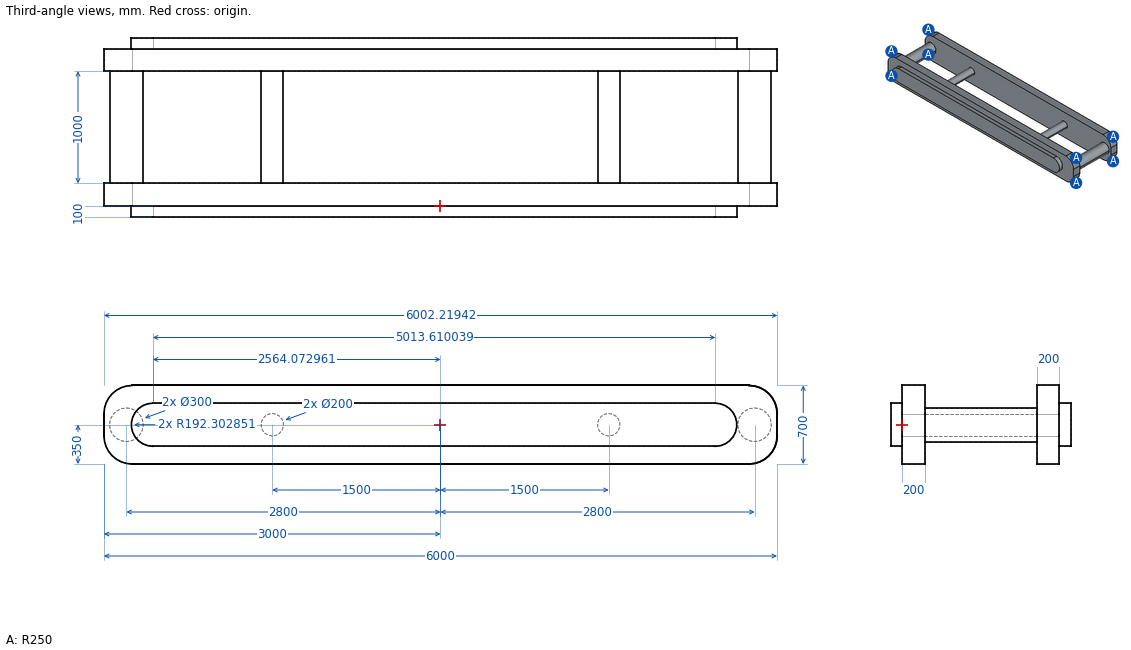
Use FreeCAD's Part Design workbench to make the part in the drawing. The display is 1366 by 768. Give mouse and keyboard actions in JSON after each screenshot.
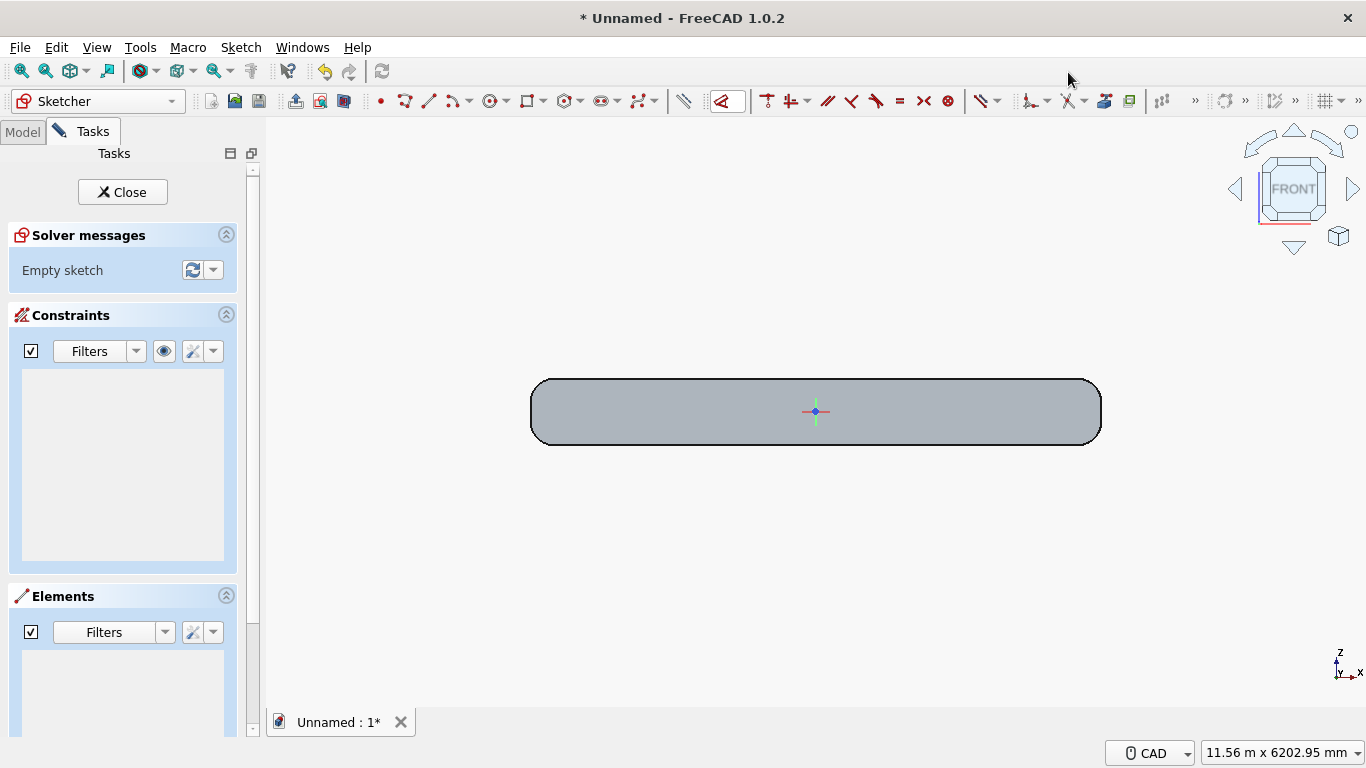
{"action": "left_click", "coordinate": [602, 102]}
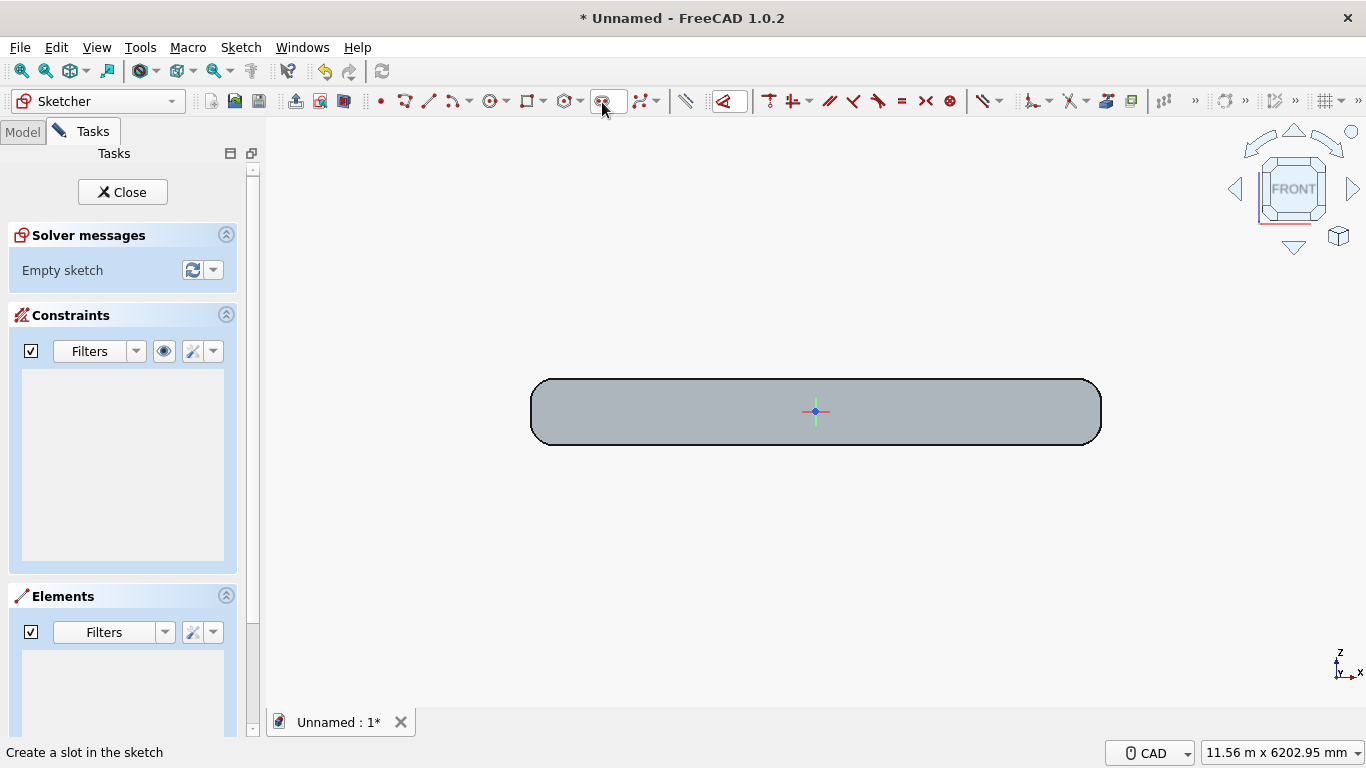
{"action": "scroll", "coordinate": [572, 412], "scroll_direction": "up", "scroll_amount": 2}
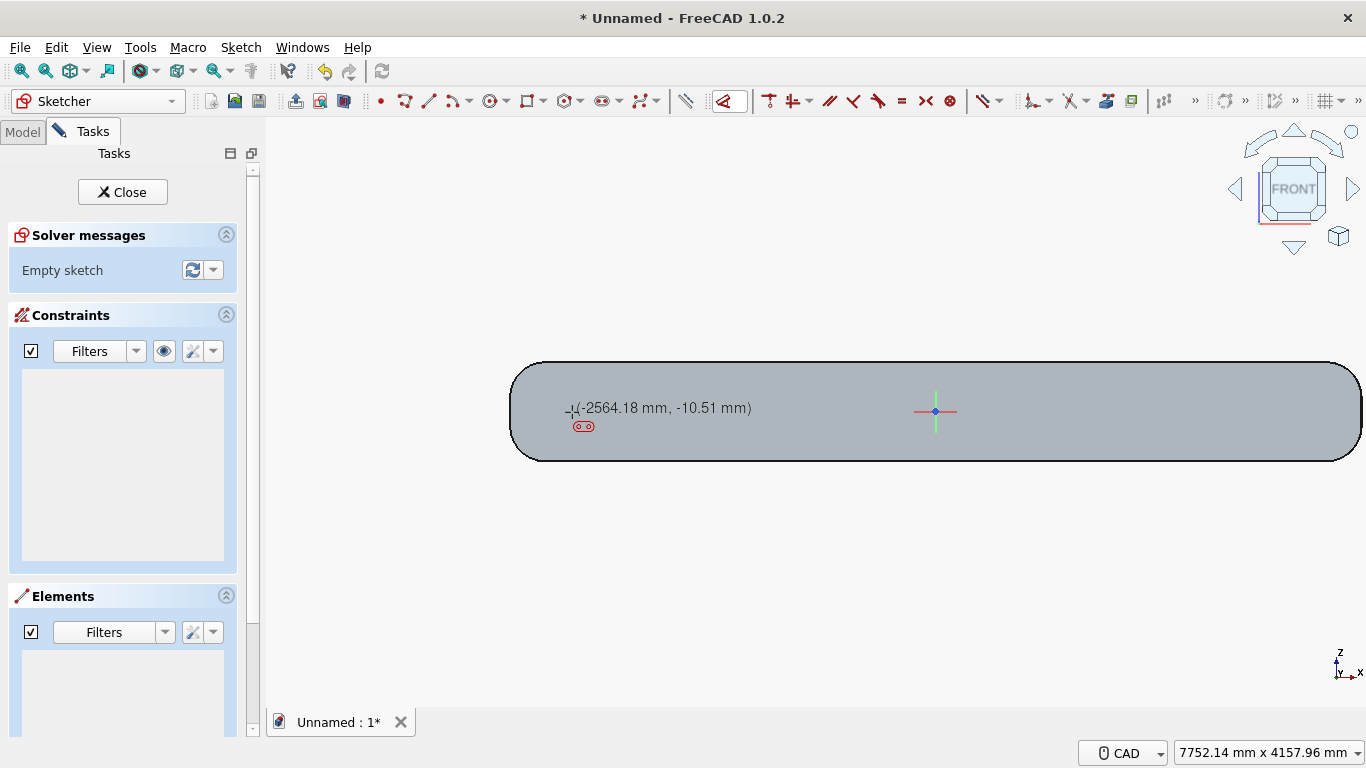
{"action": "left_click", "coordinate": [572, 412]}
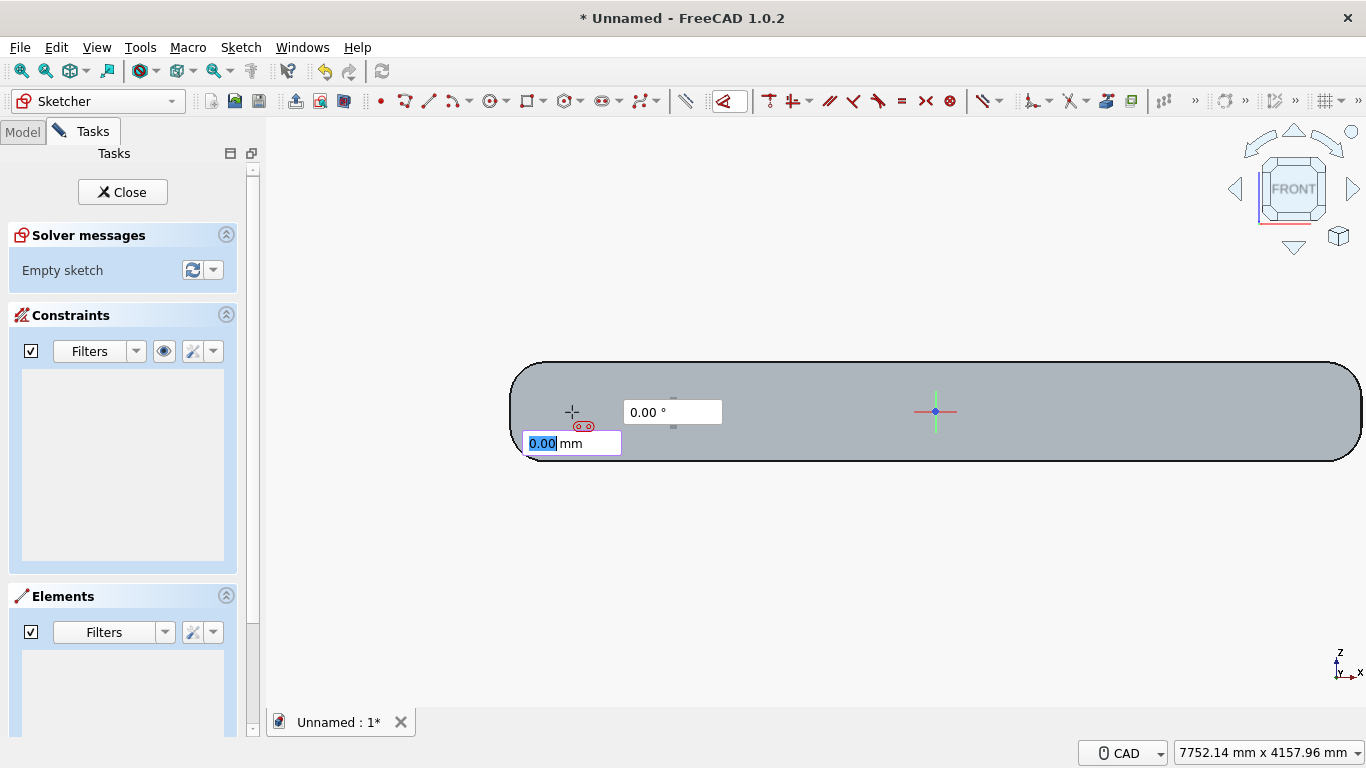
{"action": "scroll", "coordinate": [294, 413], "scroll_direction": "down", "scroll_amount": 1}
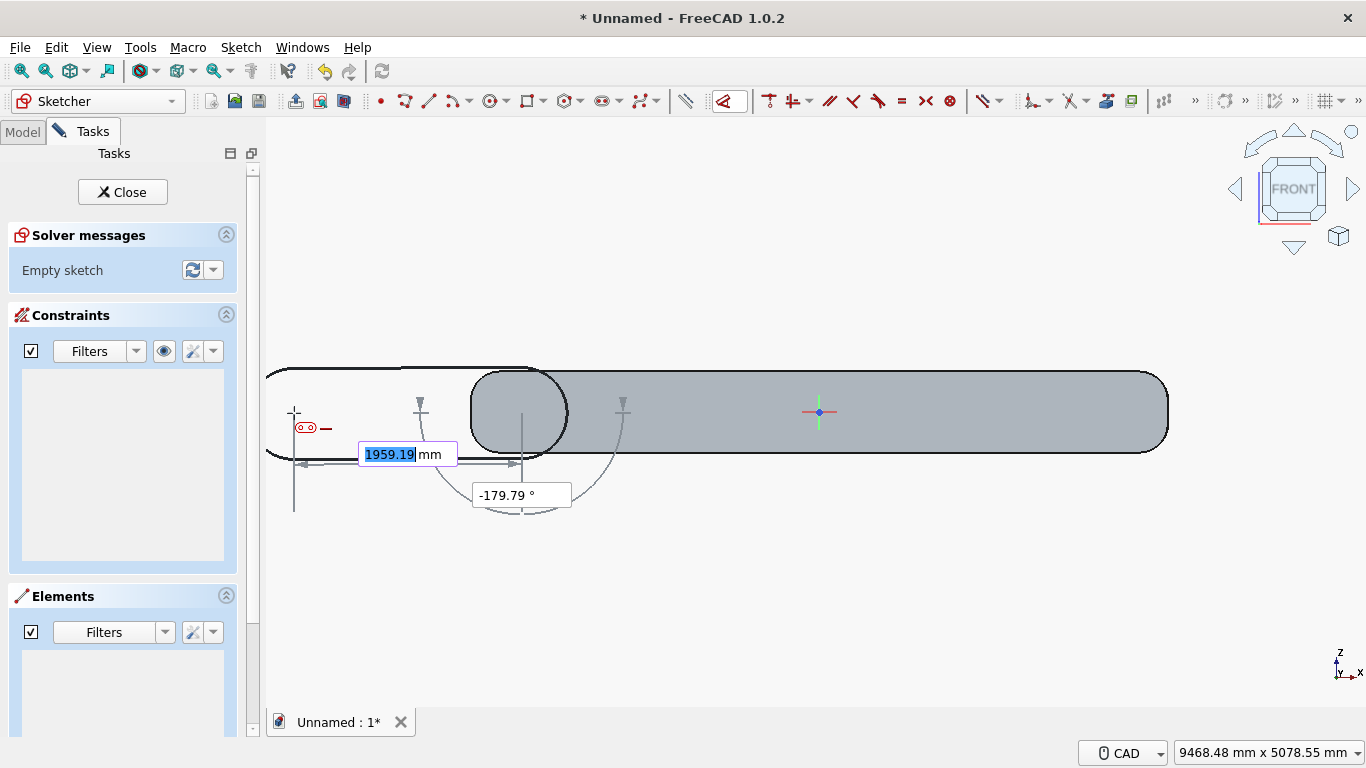
{"action": "left_click", "coordinate": [1104, 403]}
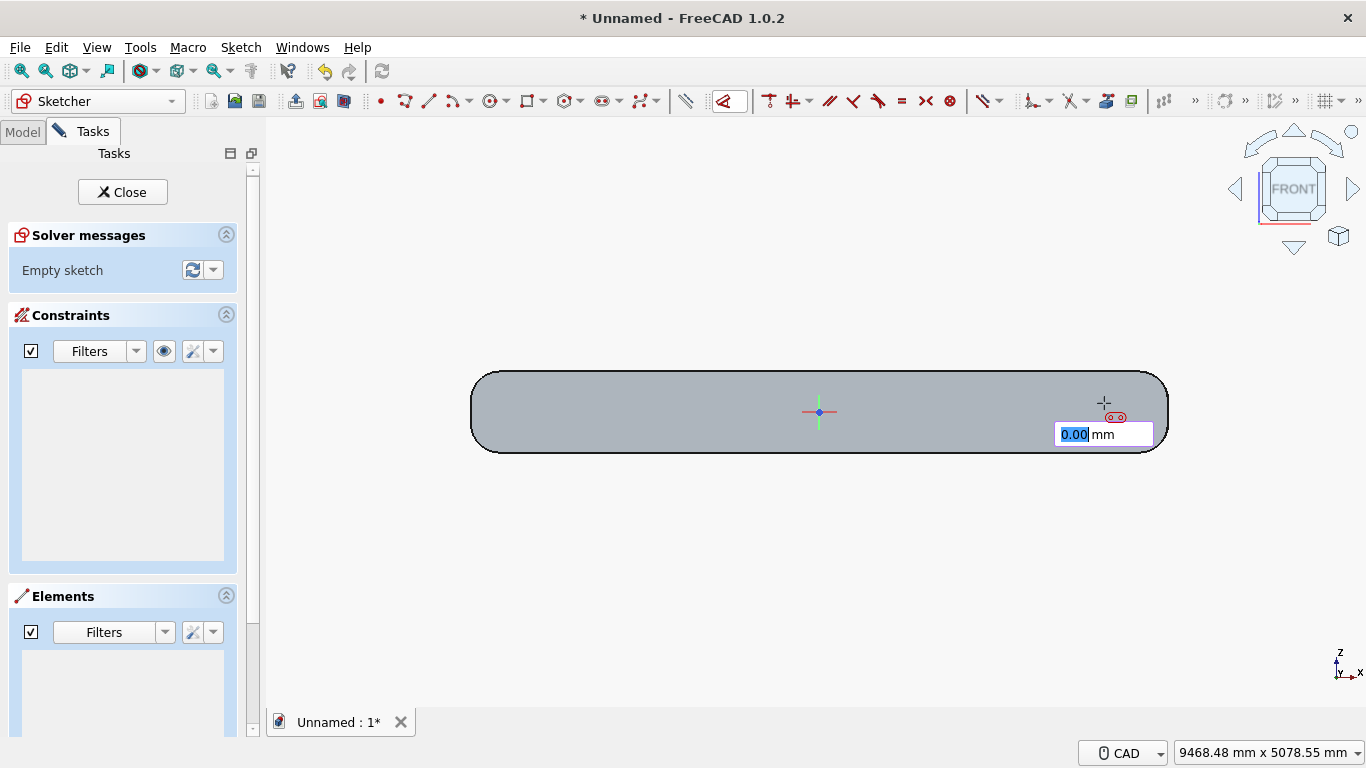
{"action": "left_click", "coordinate": [900, 390]}
{"action": "key", "text": "Escape"}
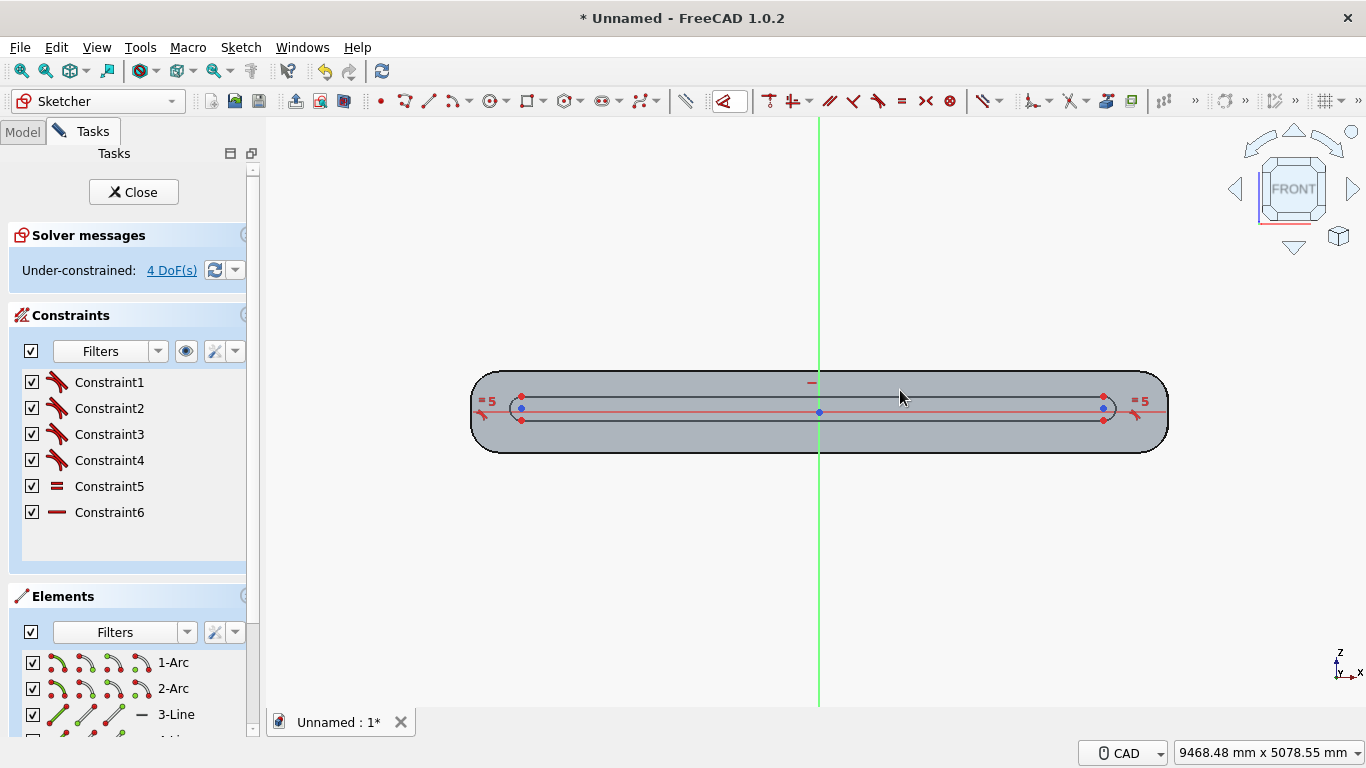
{"action": "left_click", "coordinate": [522, 409]}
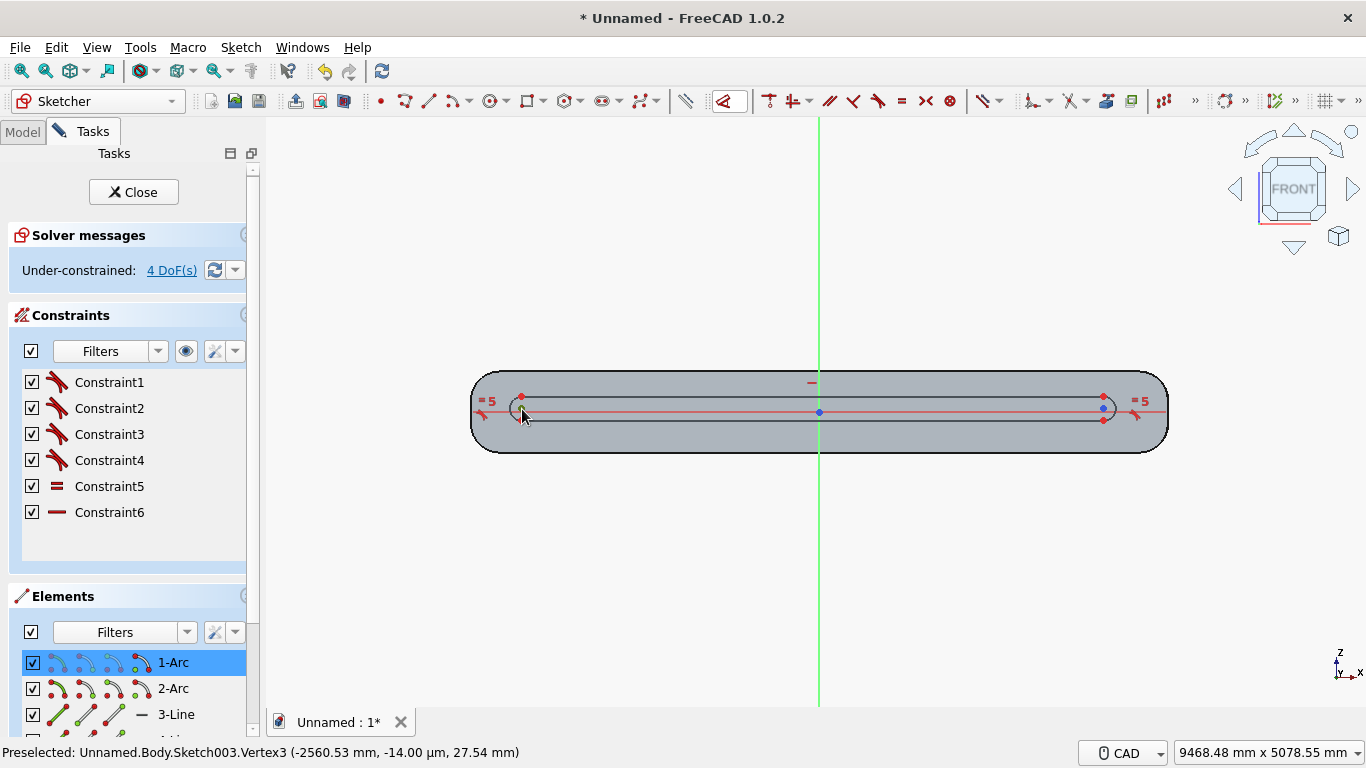
{"action": "left_click", "coordinate": [877, 412]}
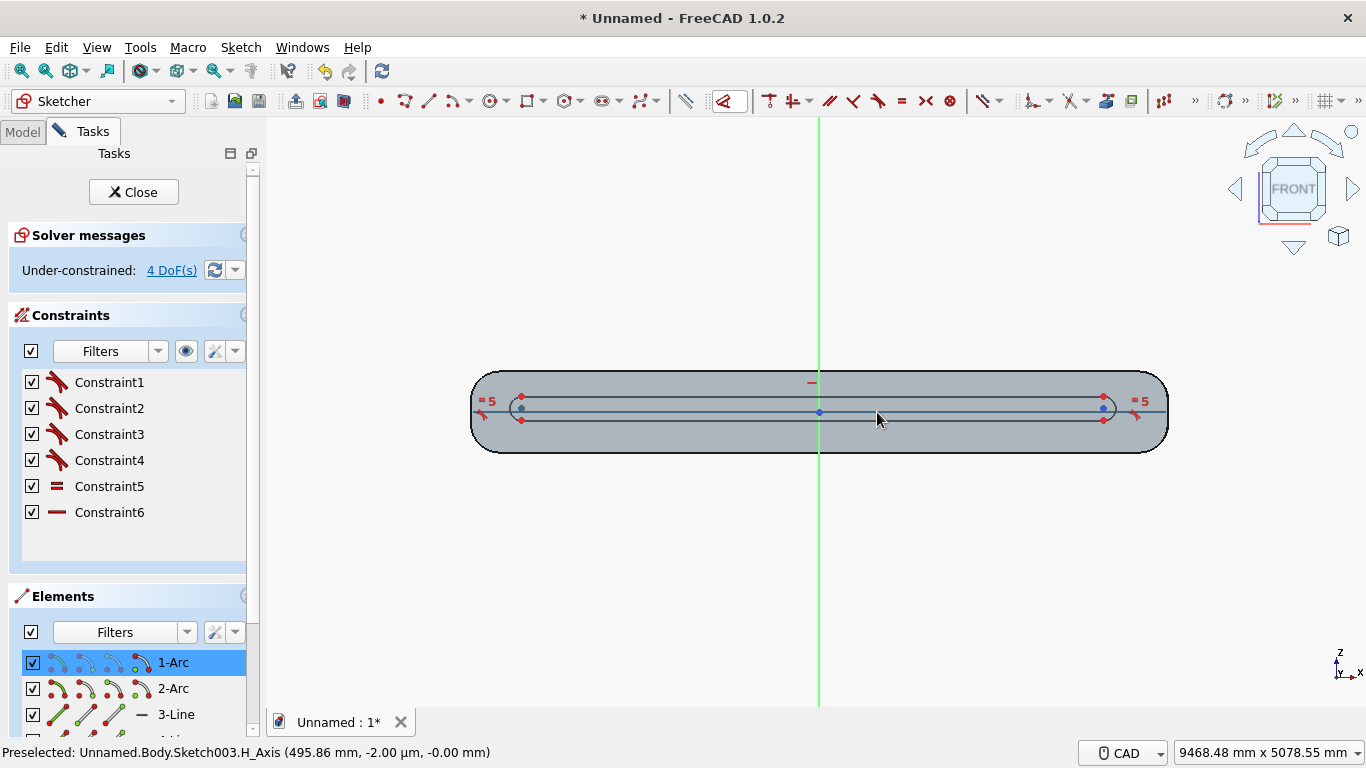
{"action": "left_click", "coordinate": [770, 102]}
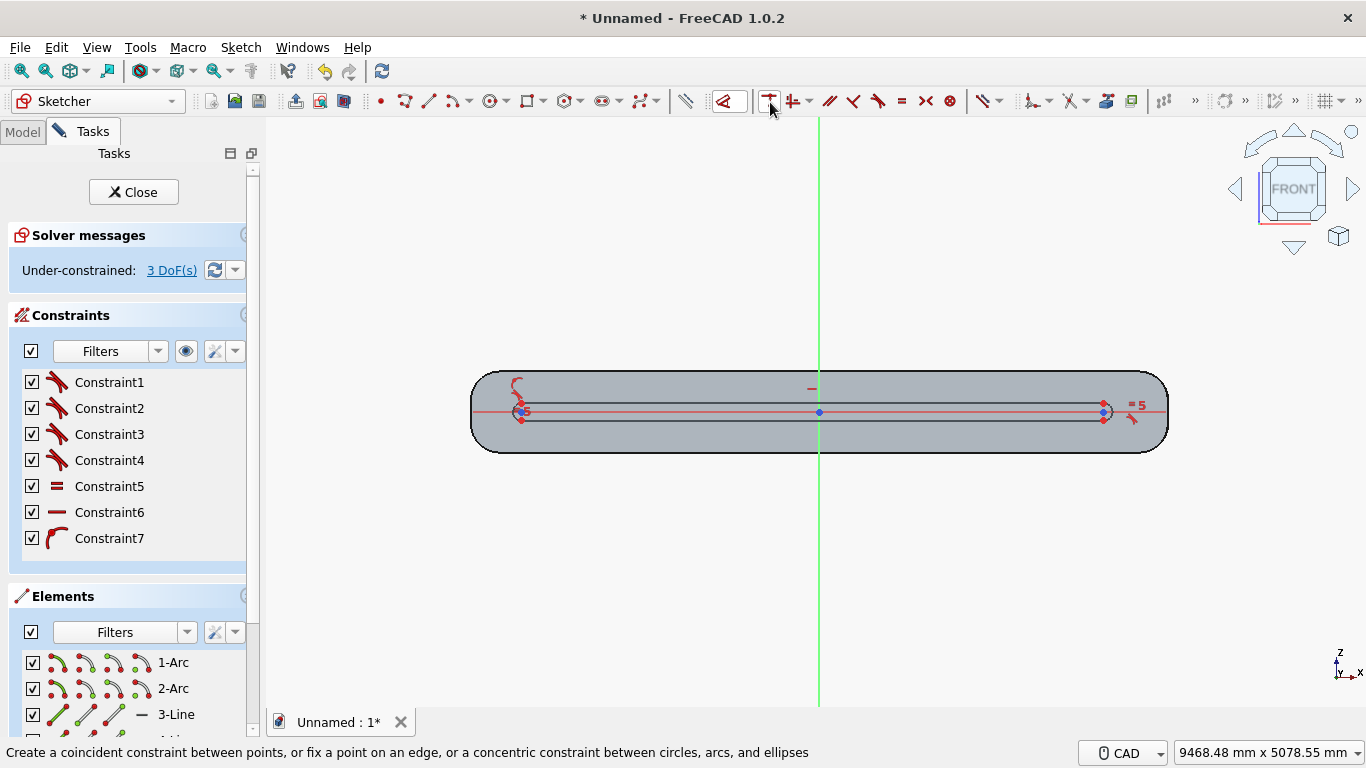
{"action": "scroll", "coordinate": [513, 412], "scroll_direction": "up", "scroll_amount": 3}